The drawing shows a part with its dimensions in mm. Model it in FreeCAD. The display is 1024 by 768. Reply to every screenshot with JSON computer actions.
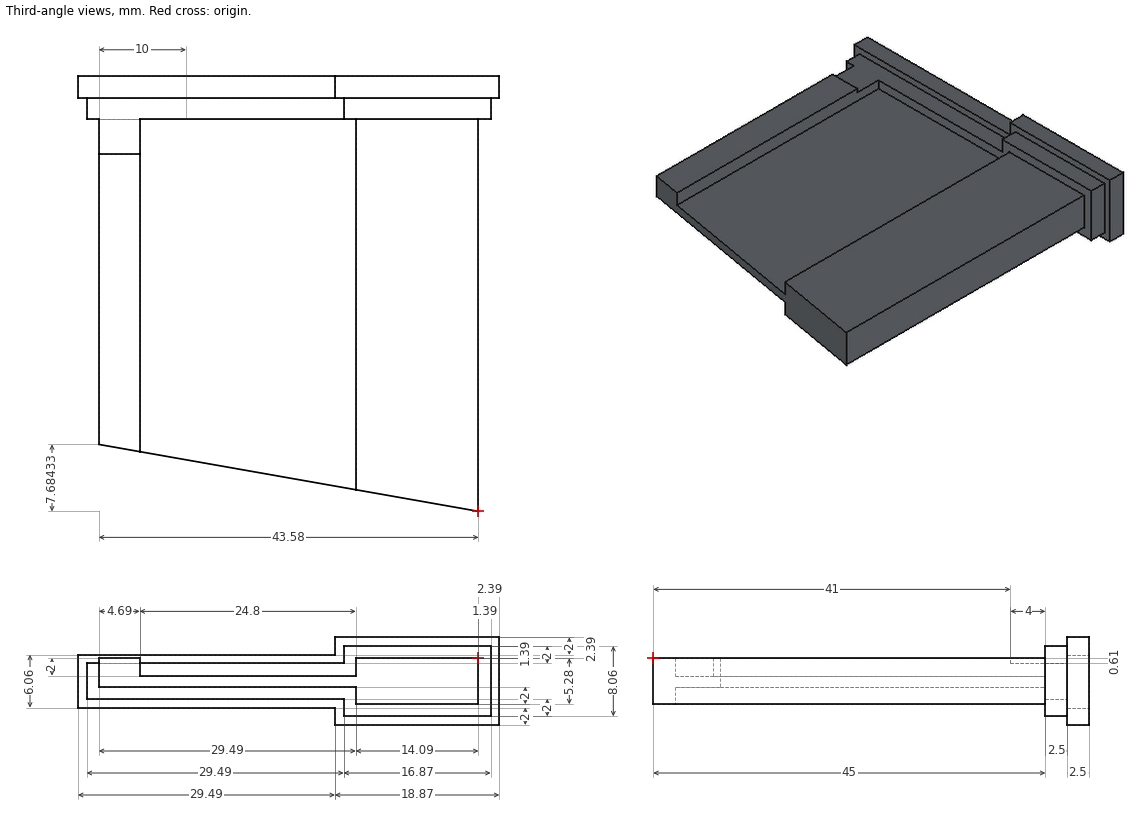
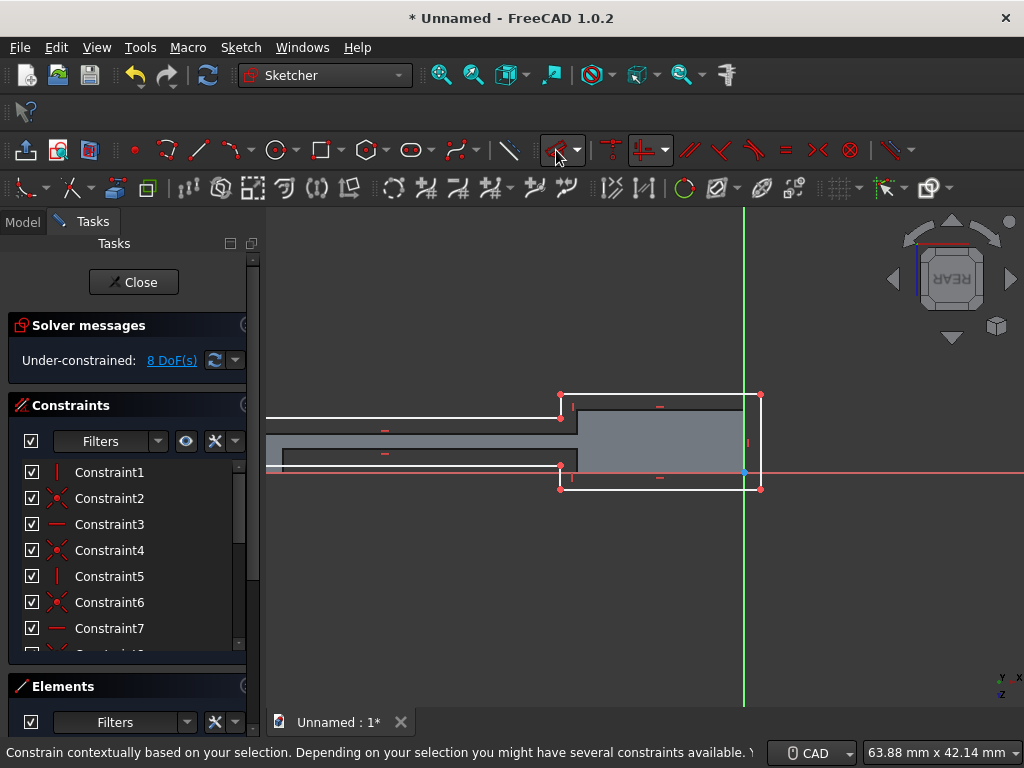
{"action": "scroll", "coordinate": [561, 404], "scroll_direction": "up", "scroll_amount": 3}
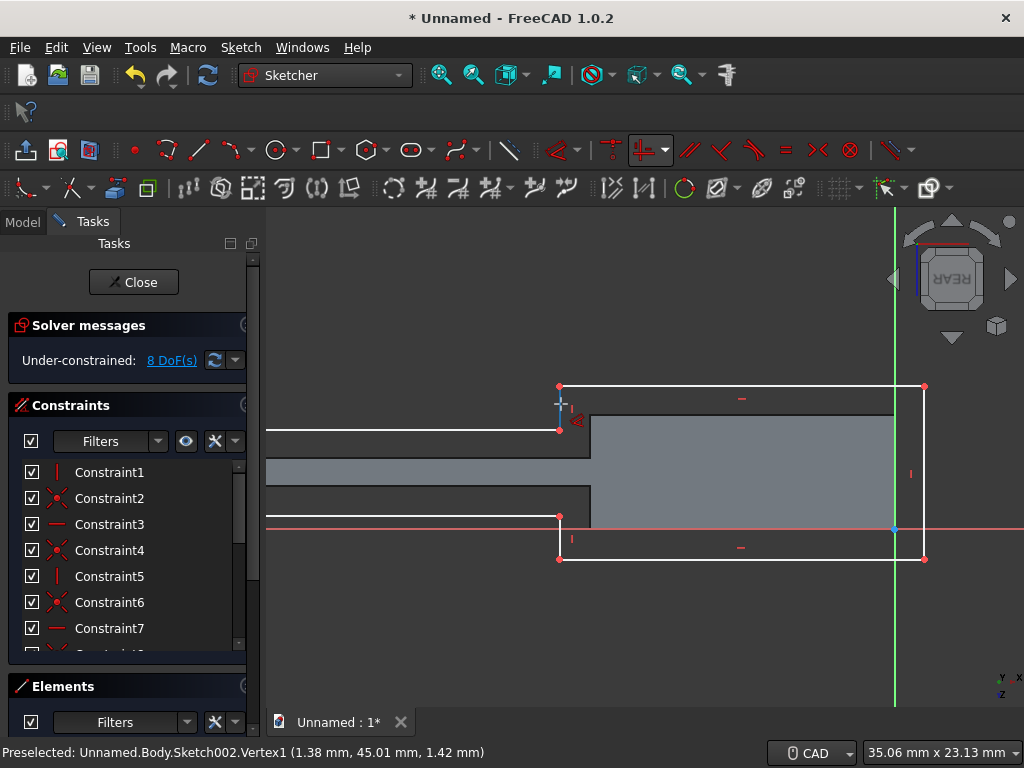
{"action": "left_click", "coordinate": [560, 404]}
{"action": "left_click", "coordinate": [594, 408]}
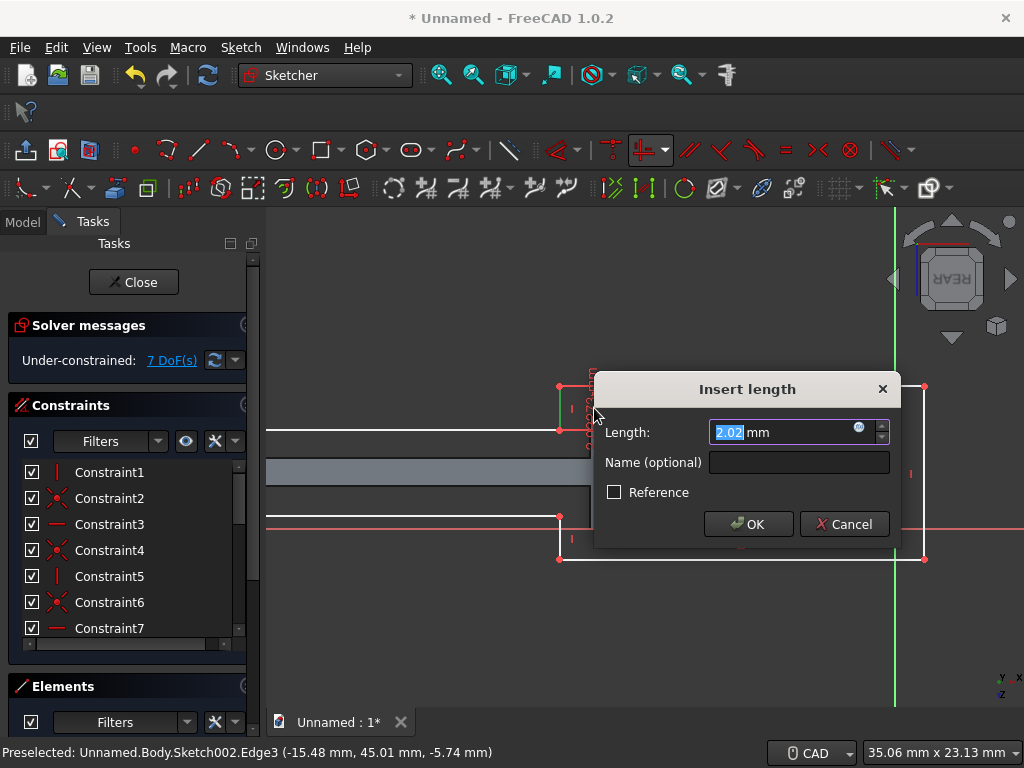
{"action": "type", "text": "2"}
{"action": "key", "text": "Return"}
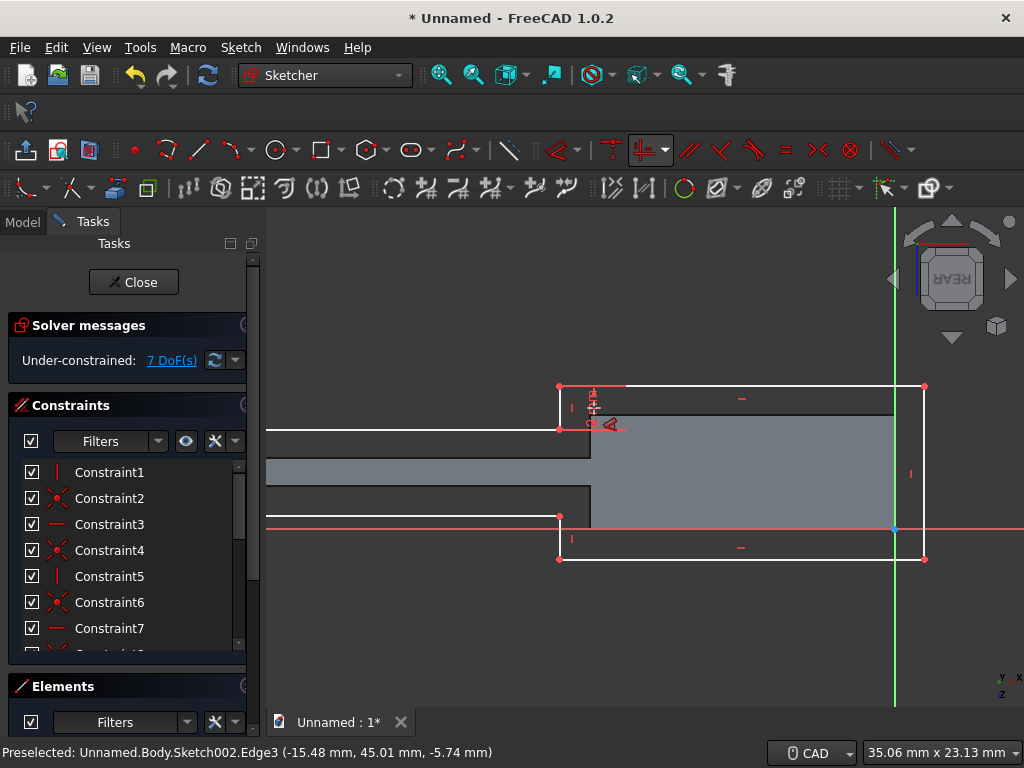
{"action": "left_click", "coordinate": [560, 529]}
{"action": "left_click", "coordinate": [526, 548]}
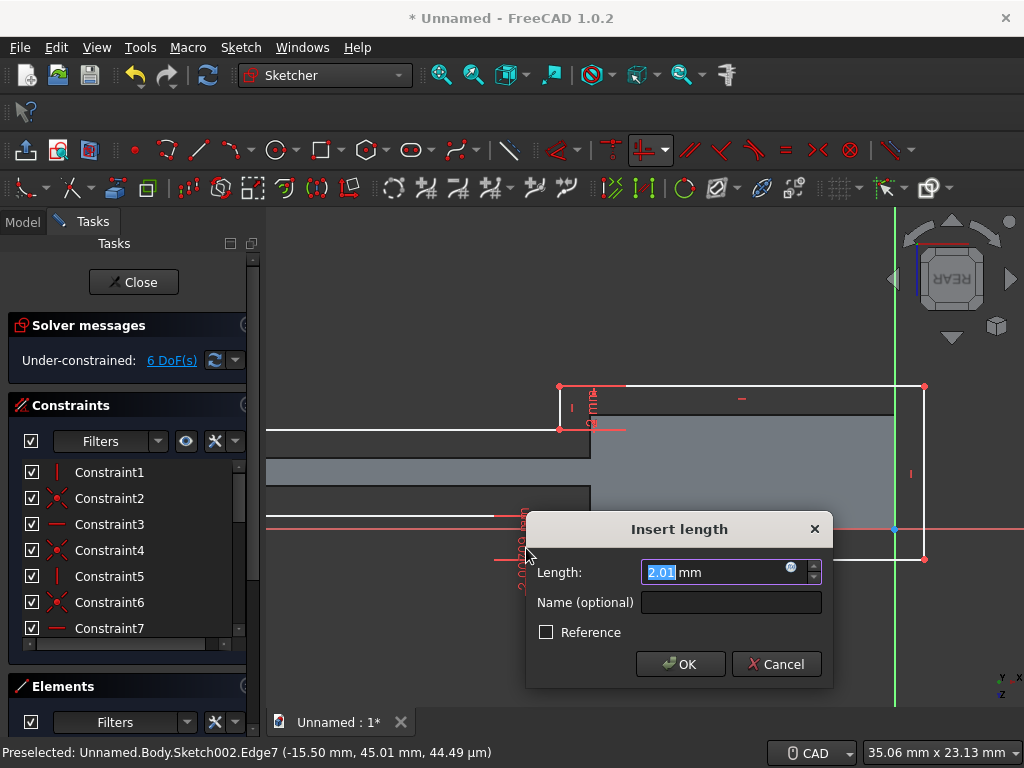
{"action": "type", "text": "2"}
{"action": "key", "text": "Return"}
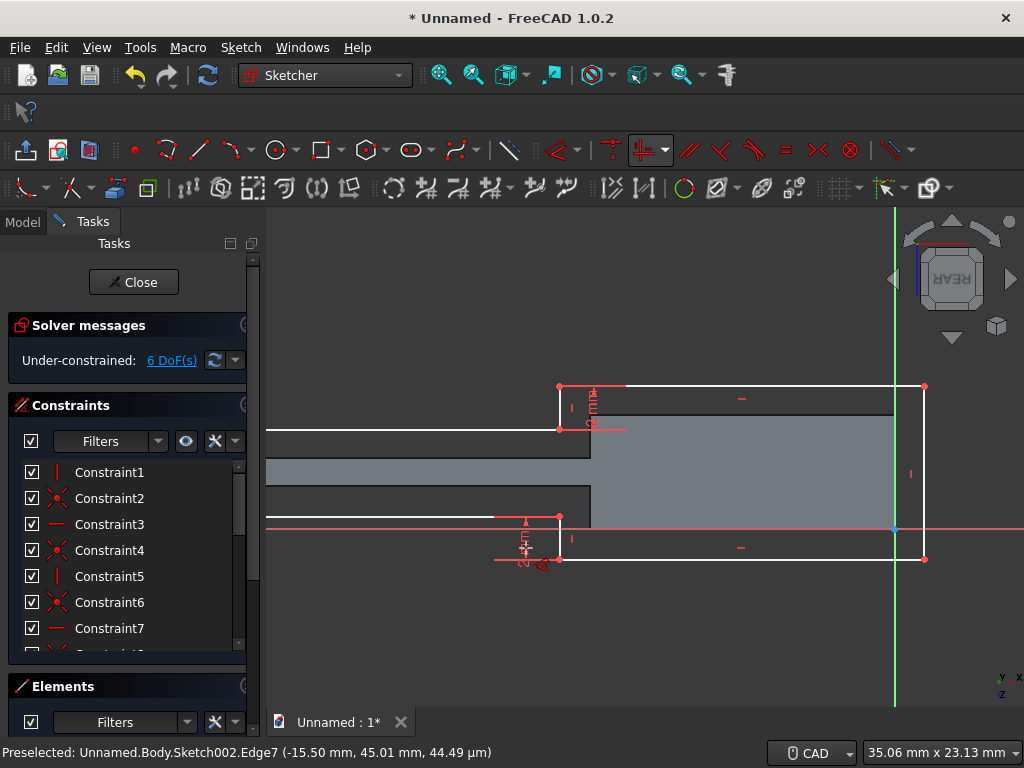
{"action": "scroll", "coordinate": [666, 448], "scroll_direction": "down", "scroll_amount": 5}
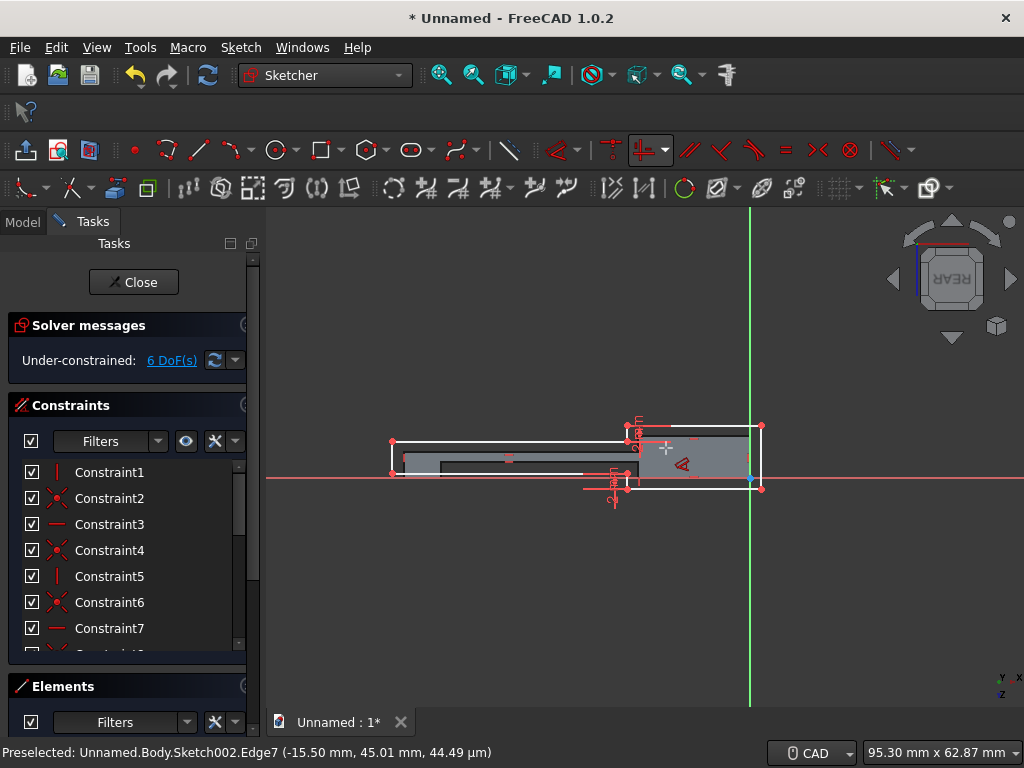
{"action": "scroll", "coordinate": [761, 470], "scroll_direction": "up", "scroll_amount": 3}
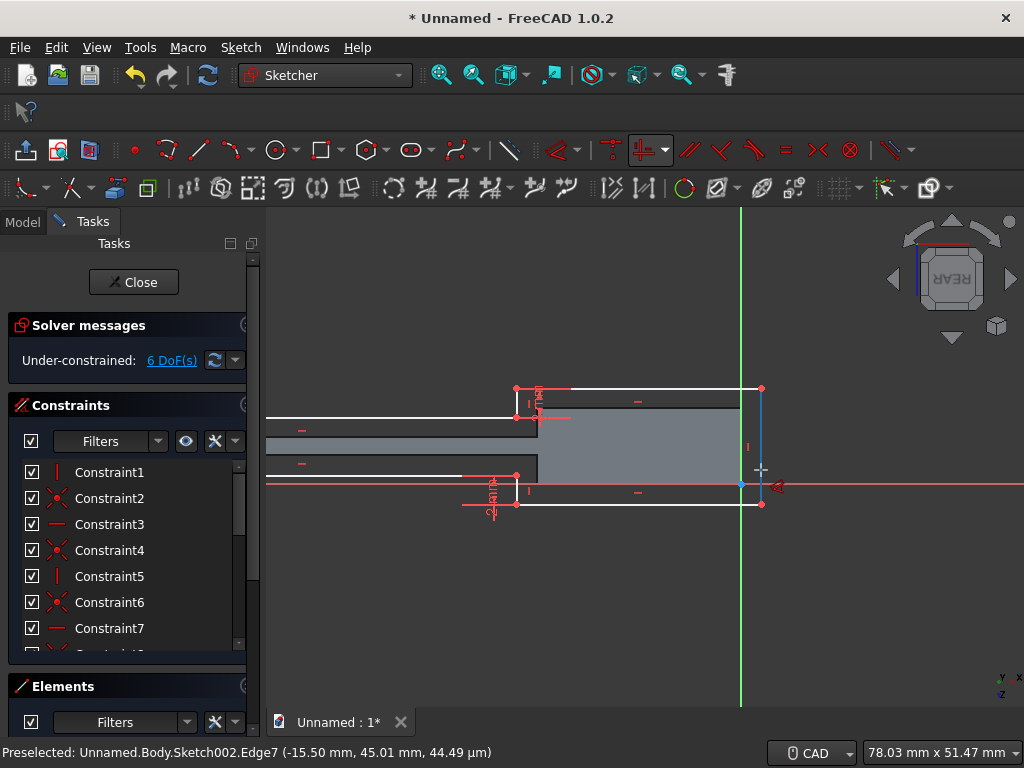
{"action": "left_click", "coordinate": [761, 470]}
{"action": "left_click", "coordinate": [795, 447]}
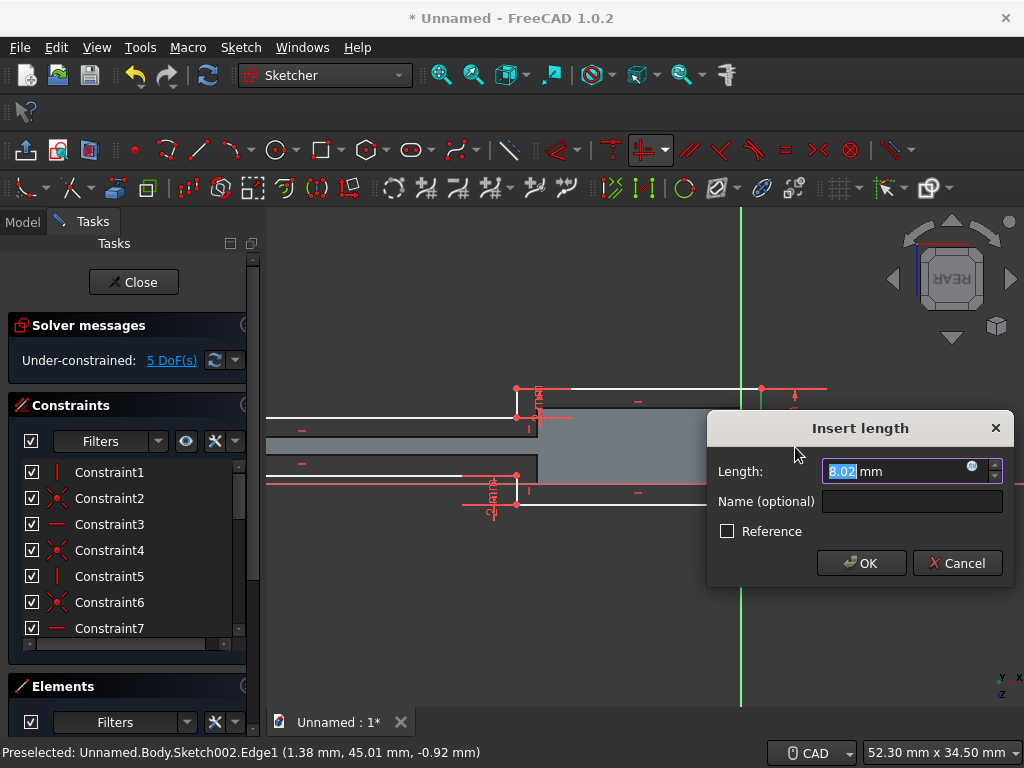
{"action": "type", "text": "8.06"}
{"action": "key", "text": "Return"}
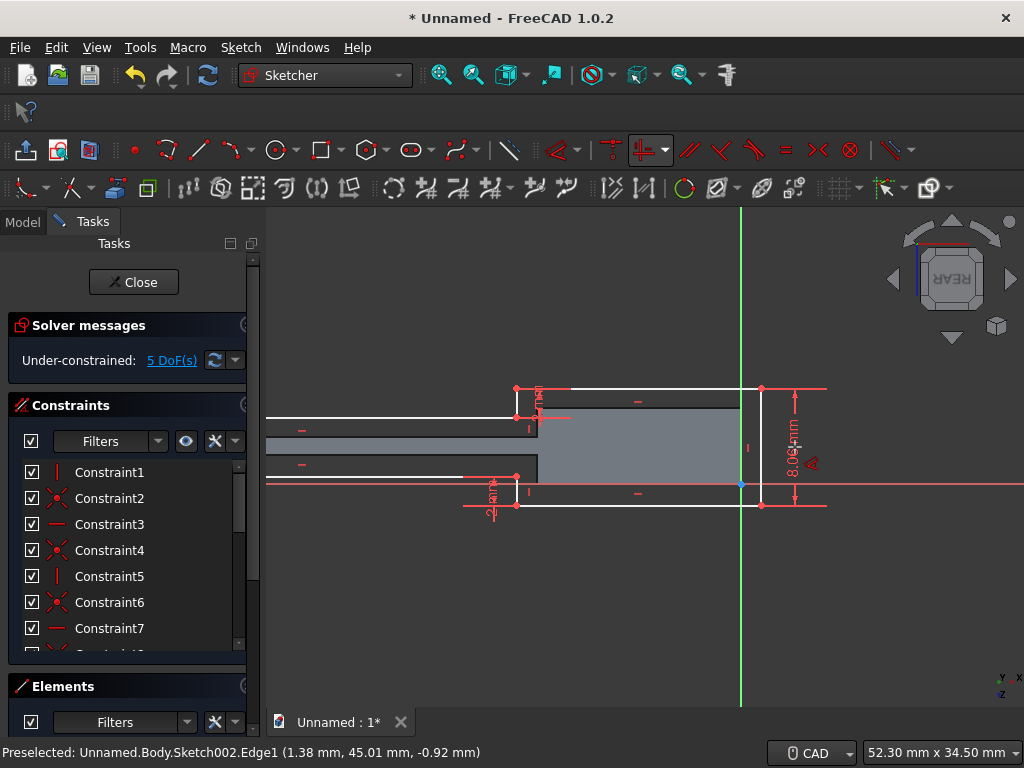
{"action": "left_click", "coordinate": [688, 389]}
{"action": "left_click", "coordinate": [639, 355]}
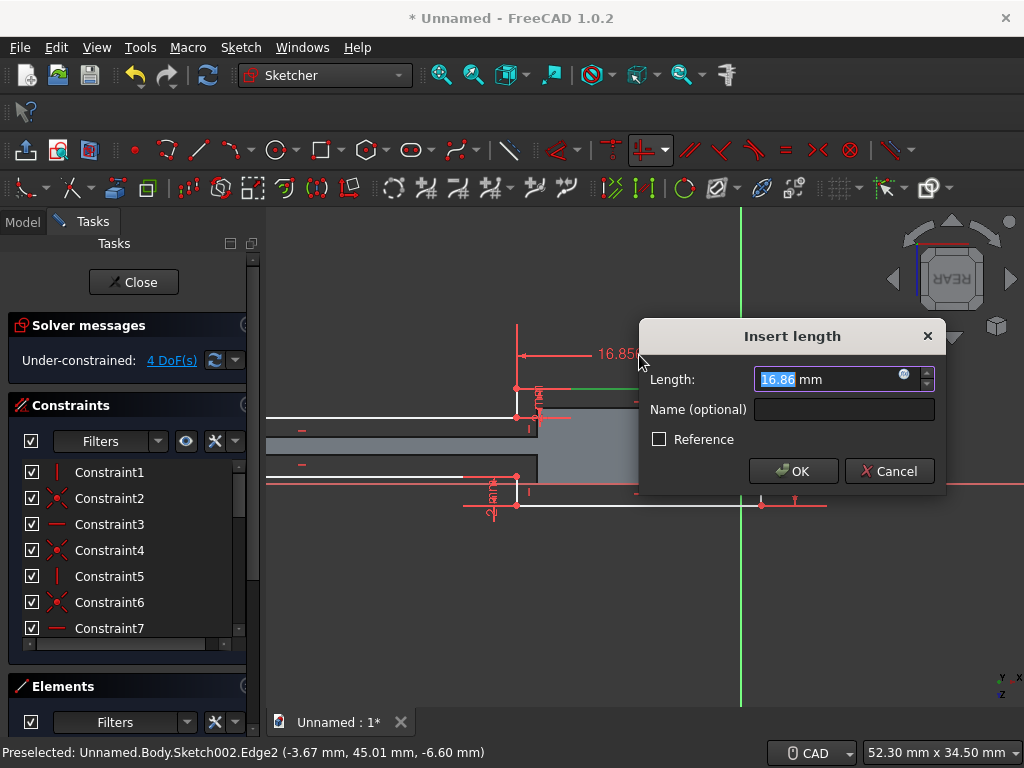
{"action": "type", "text": "16.87"}
{"action": "key", "text": "Return"}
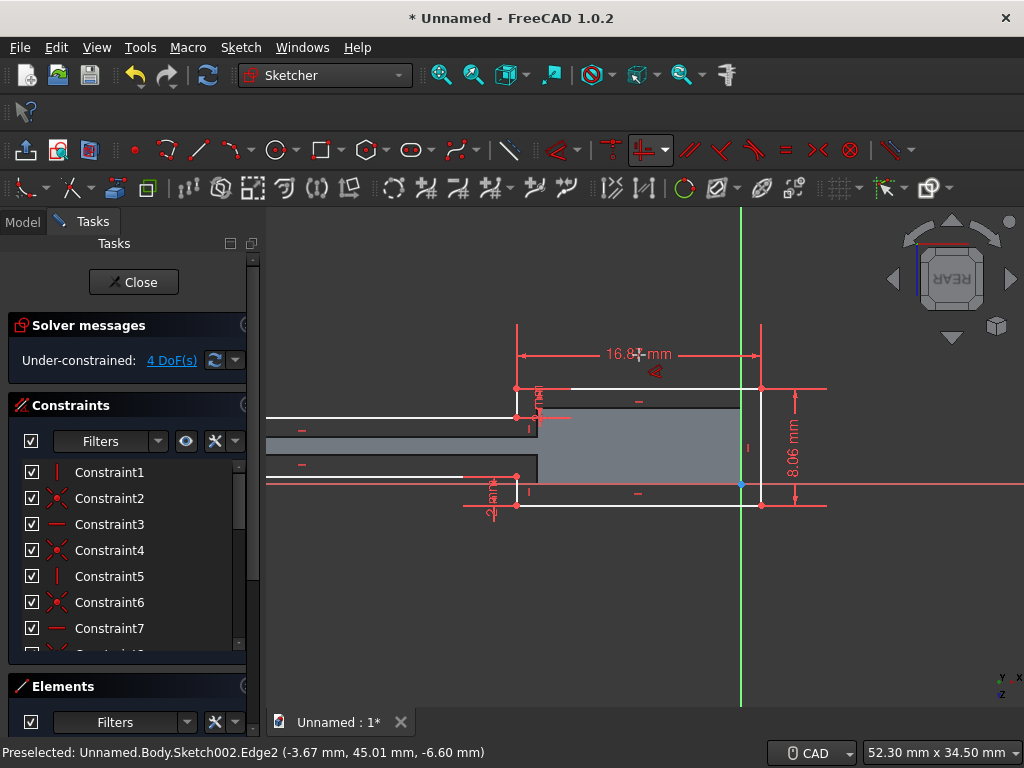
{"action": "left_click", "coordinate": [388, 418]}
{"action": "left_click", "coordinate": [405, 384]}